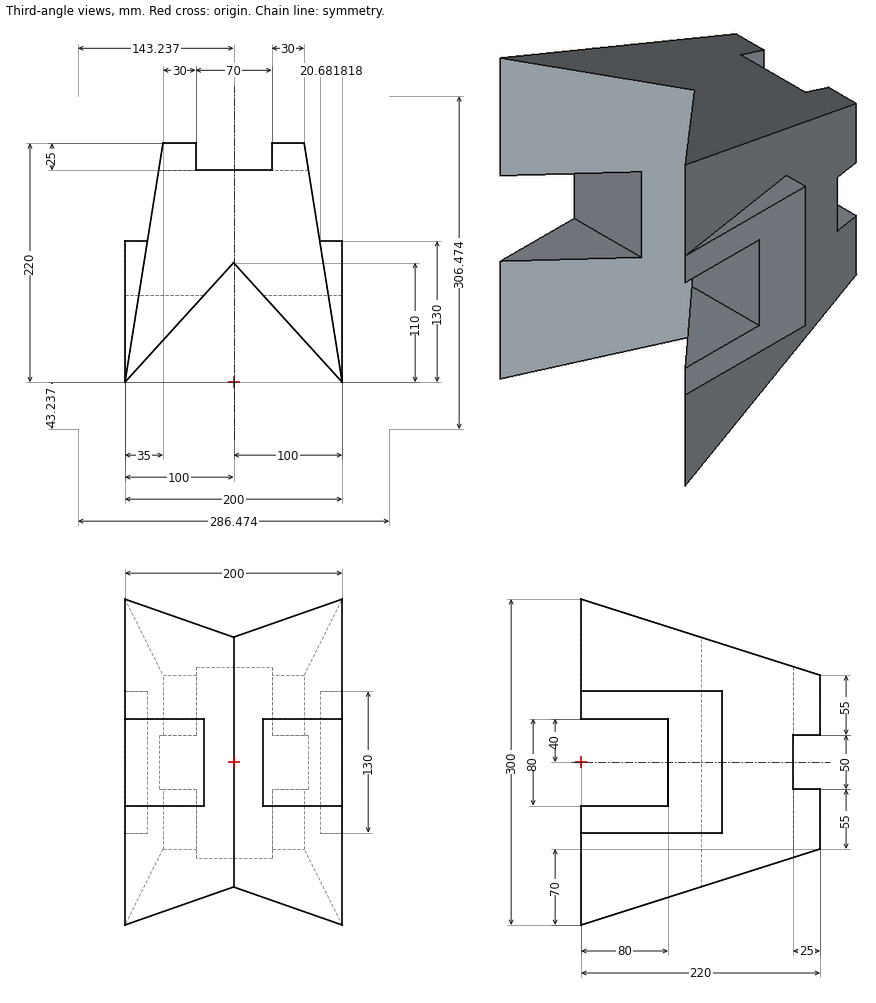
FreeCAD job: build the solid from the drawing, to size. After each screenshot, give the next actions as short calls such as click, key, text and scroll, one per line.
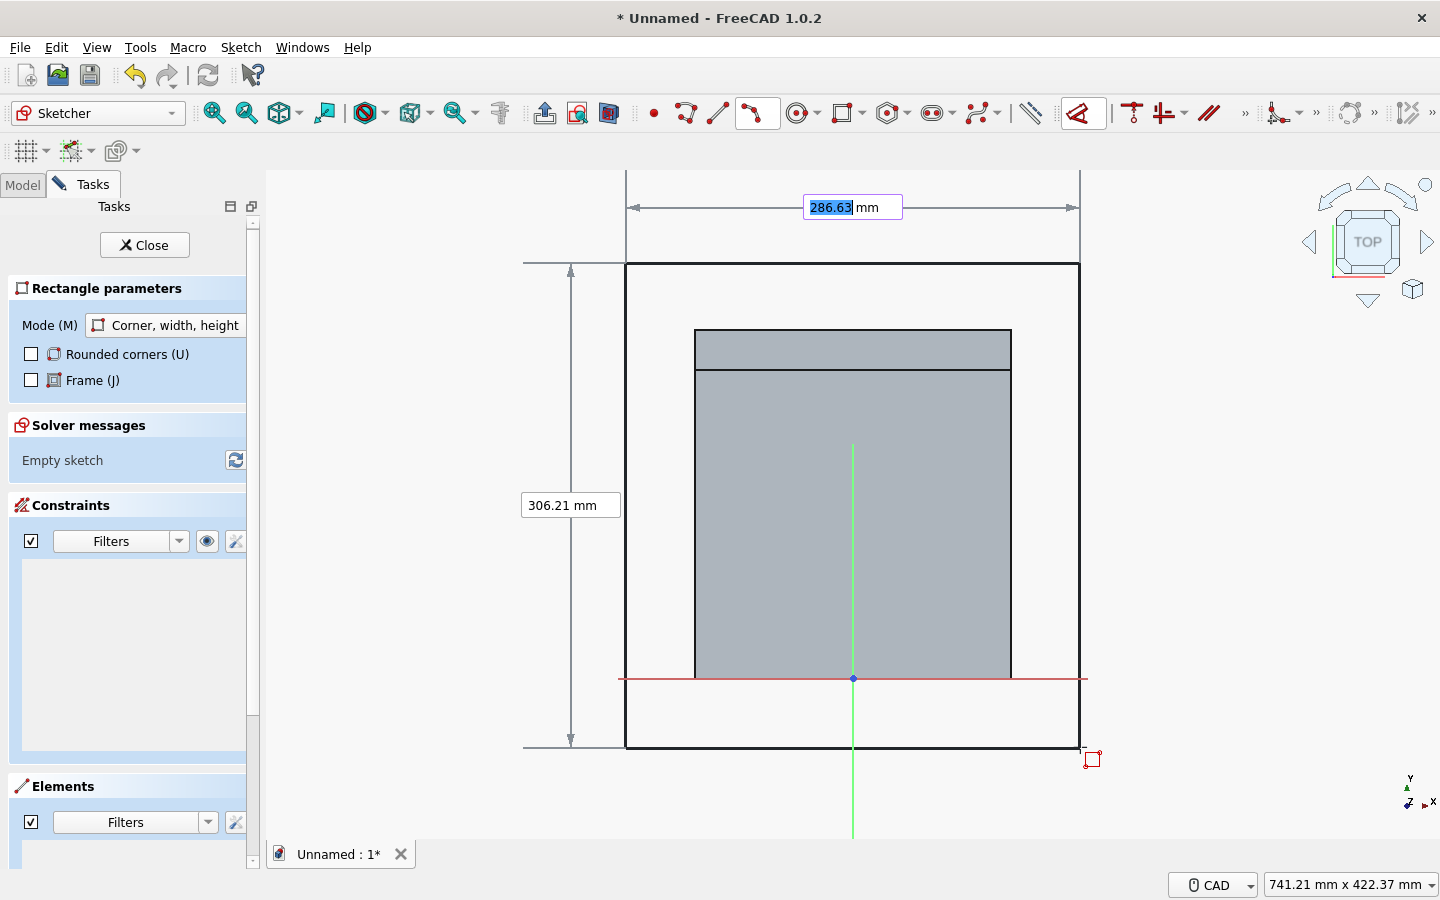
text(286.474)
key(Tab)
text(306.474)
key(Return)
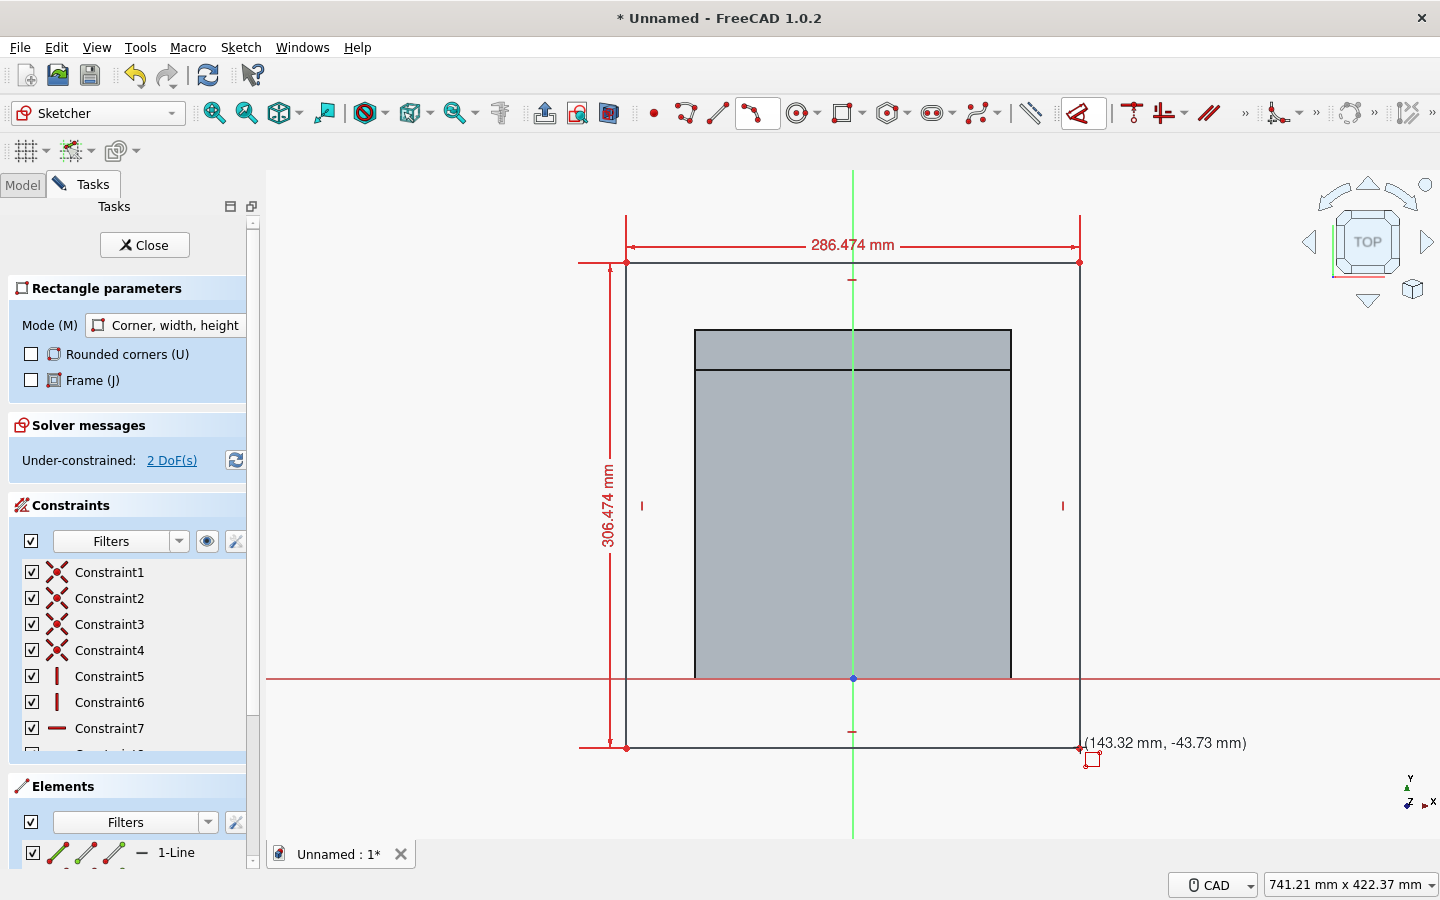
key(g)
key(m)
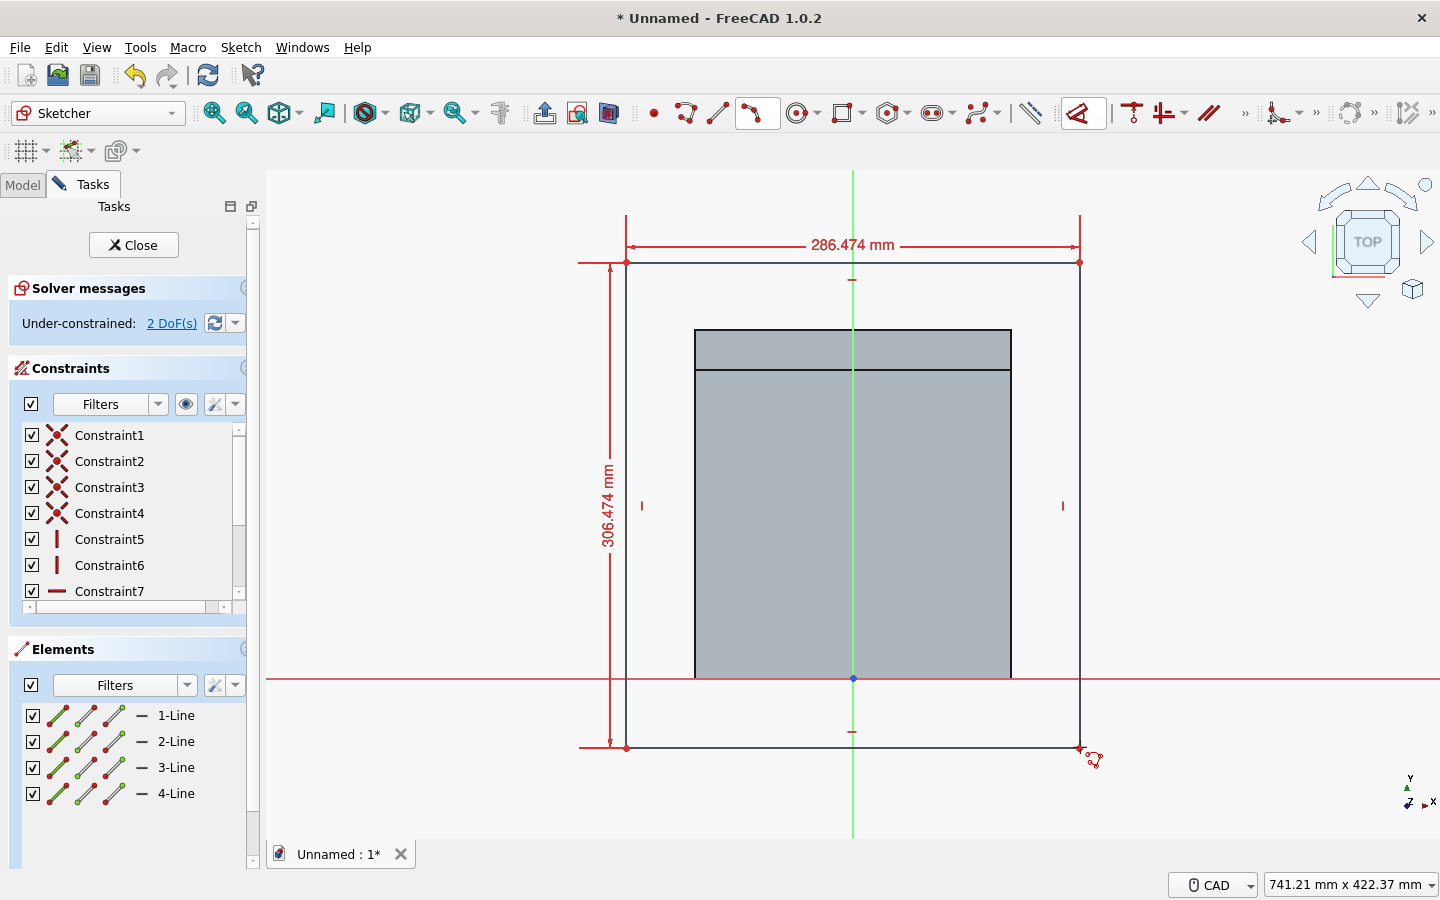
click(1011, 679)
click(695, 670)
click(750, 330)
click(798, 330)
click(798, 370)
click(908, 370)
click(908, 330)
click(956, 330)
click(1011, 679)
key(Escape)
key(Escape)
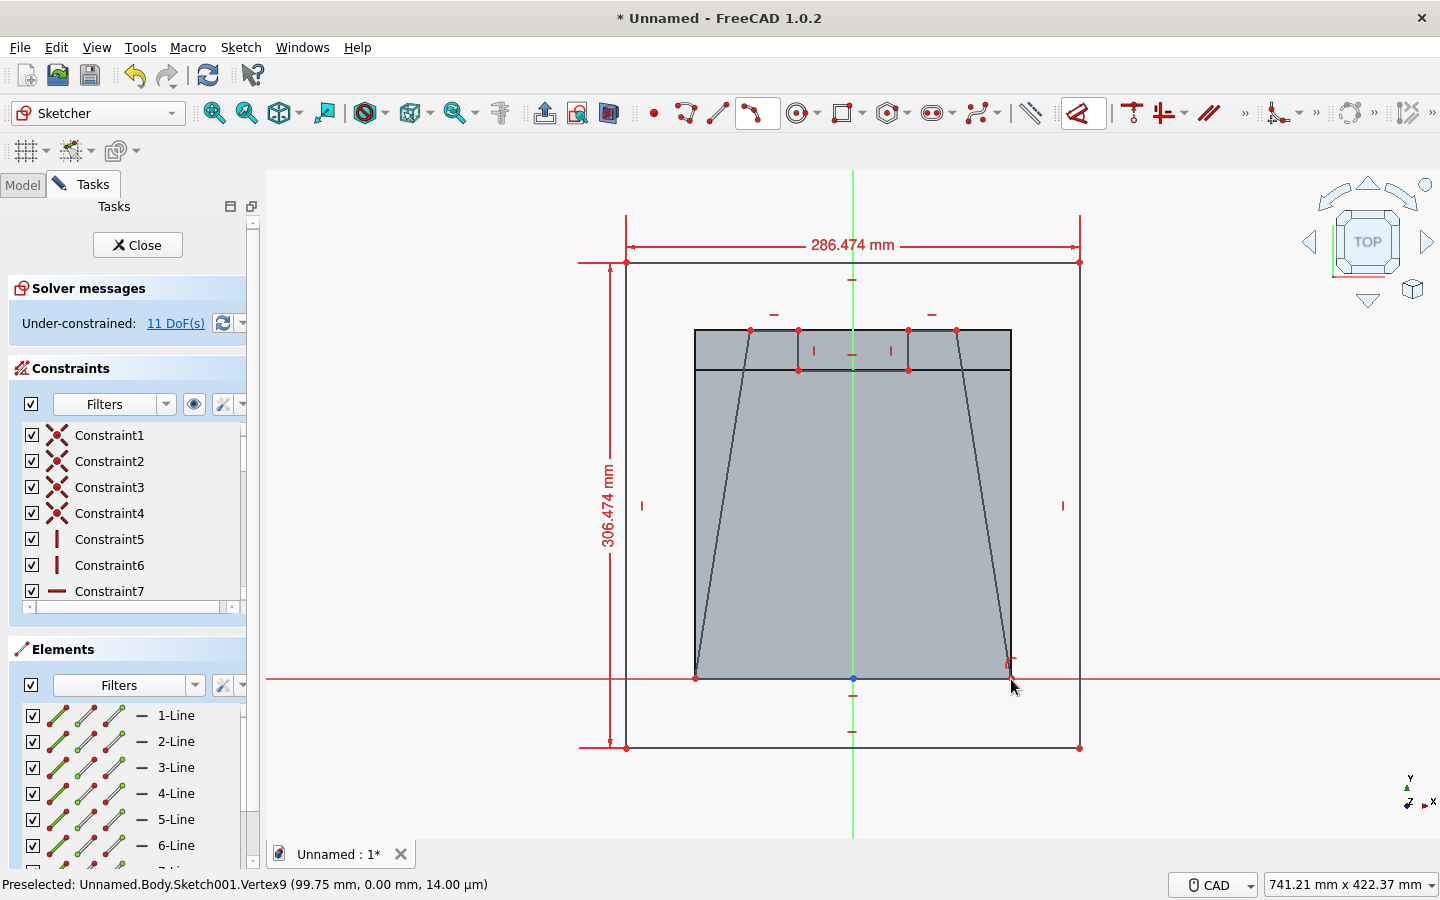
click(798, 331)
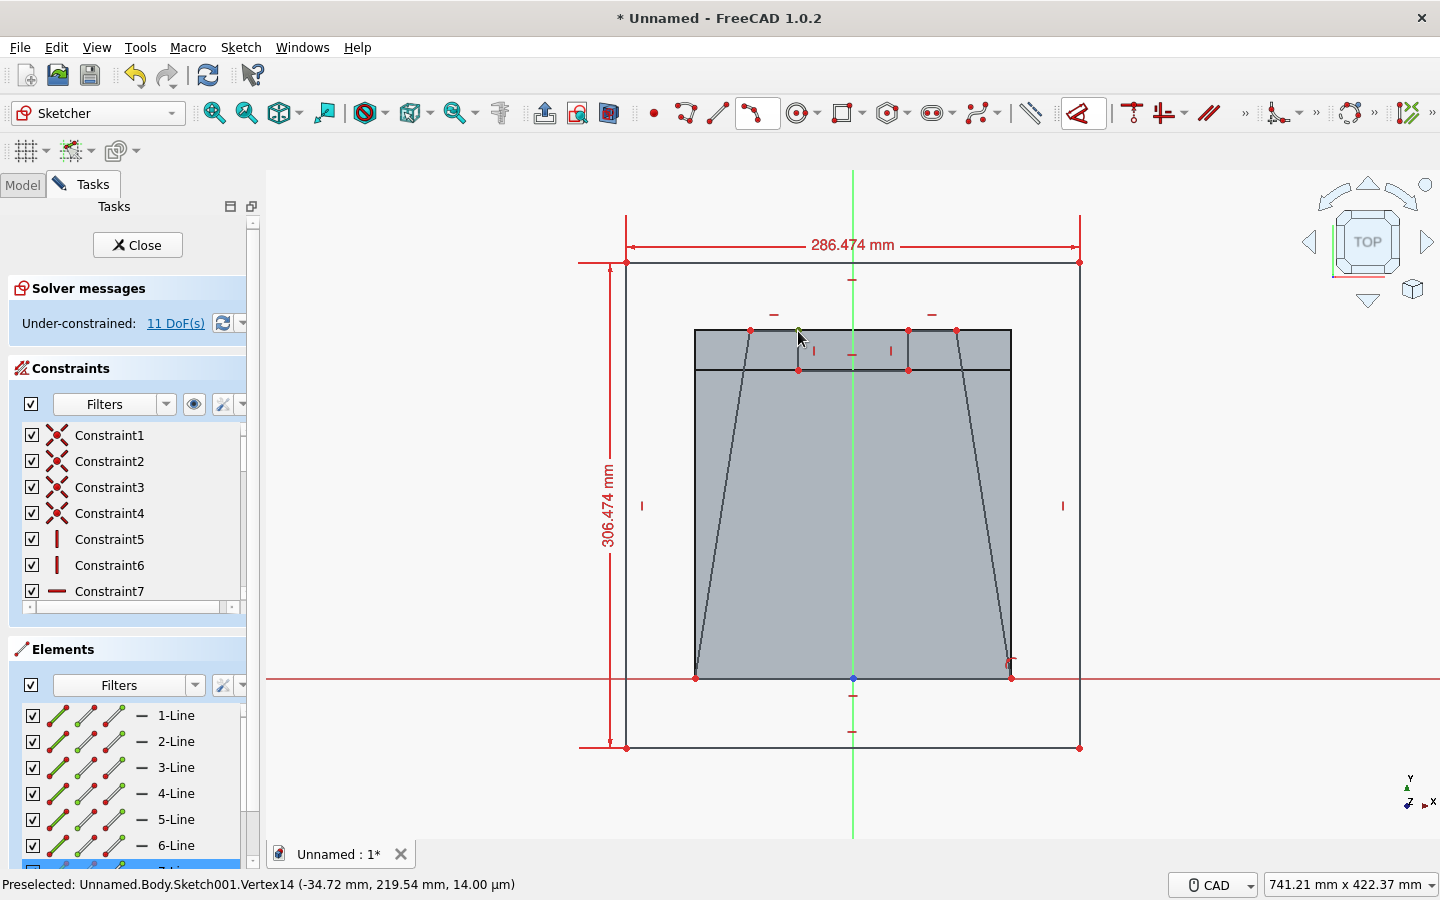
click(908, 331)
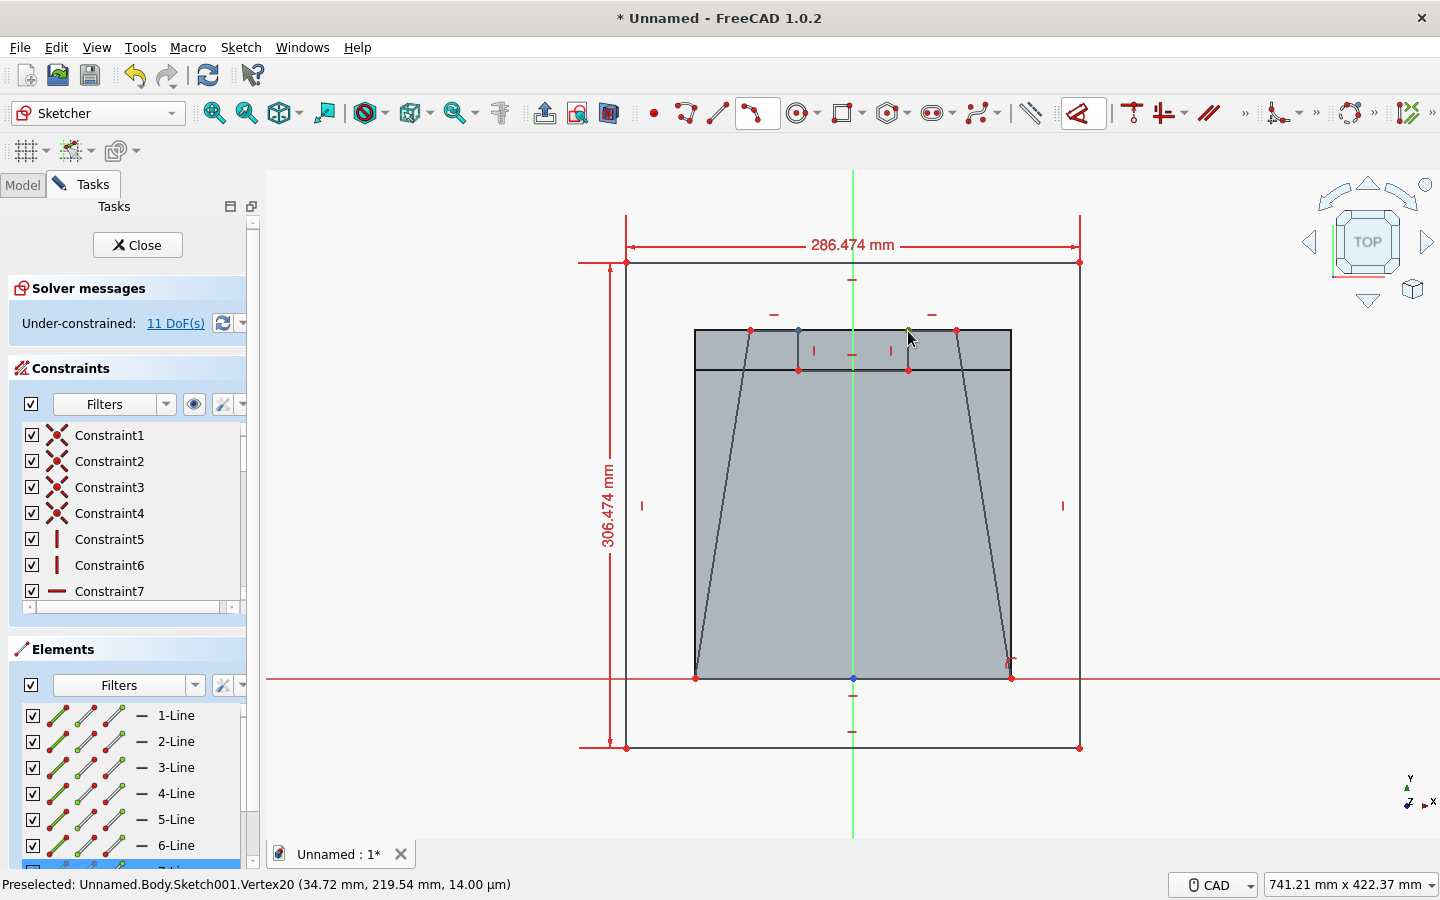
click(853, 636)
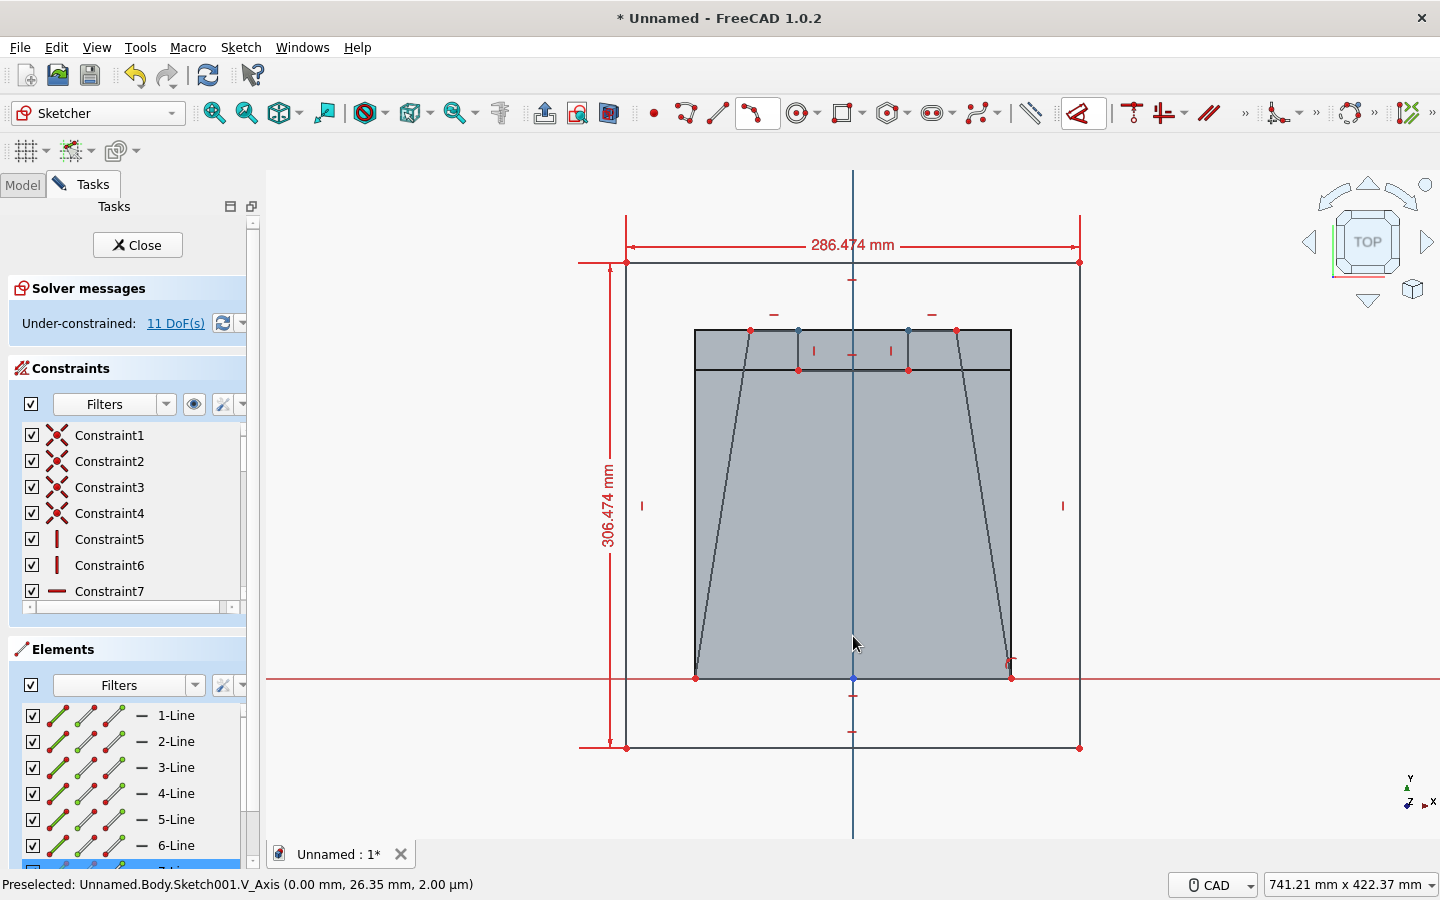
key(s)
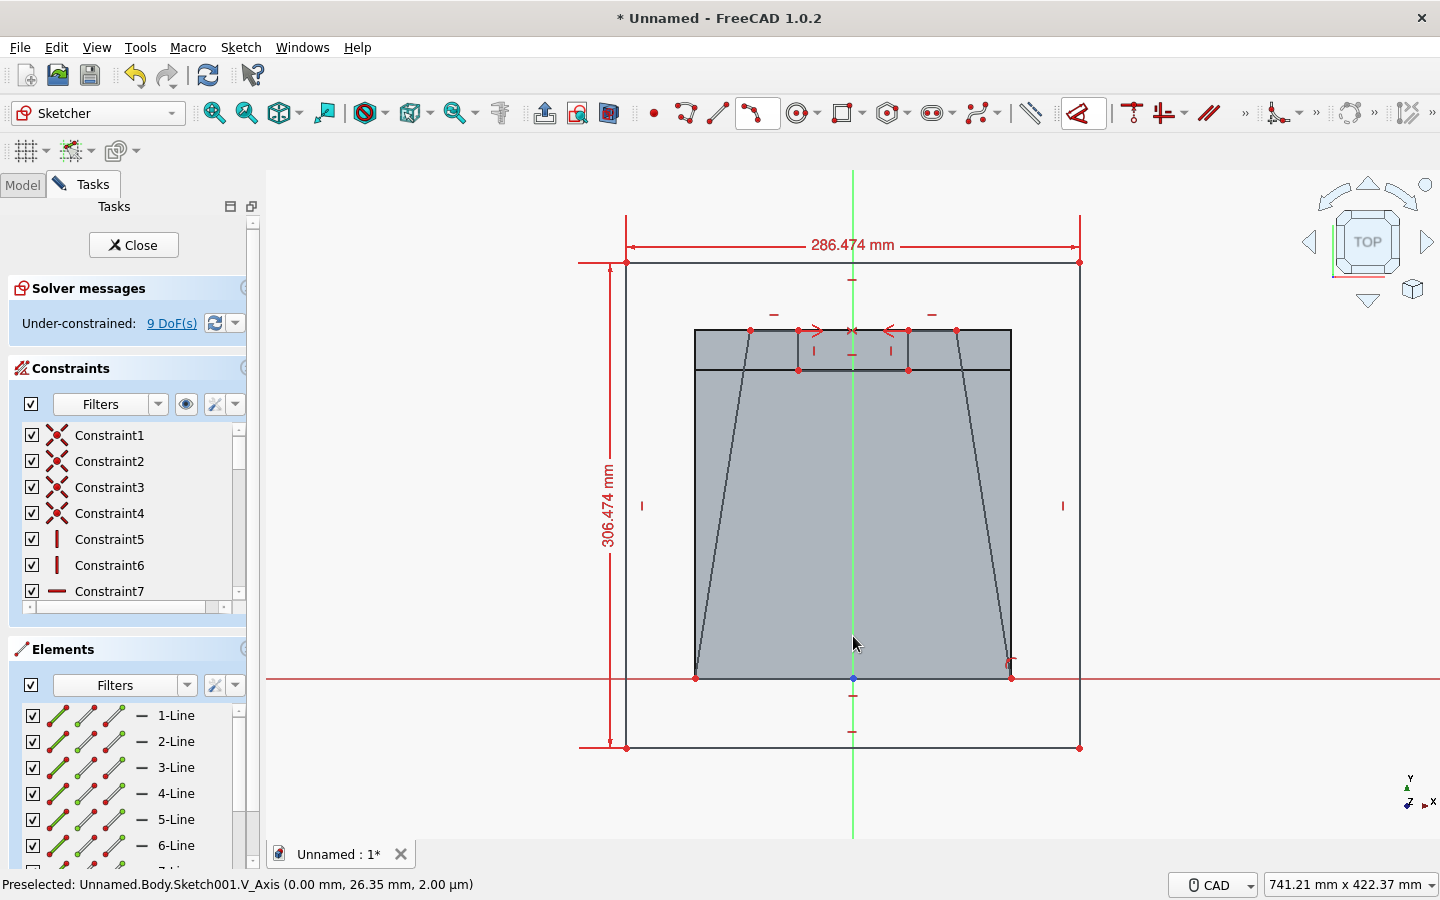
click(764, 331)